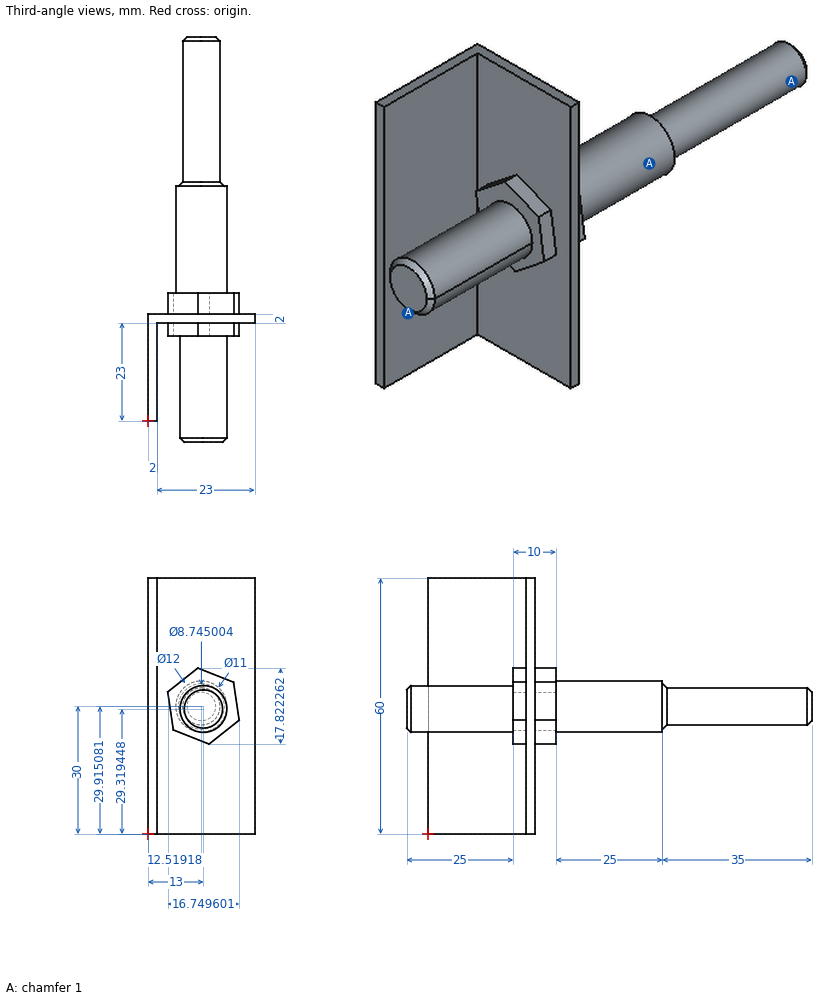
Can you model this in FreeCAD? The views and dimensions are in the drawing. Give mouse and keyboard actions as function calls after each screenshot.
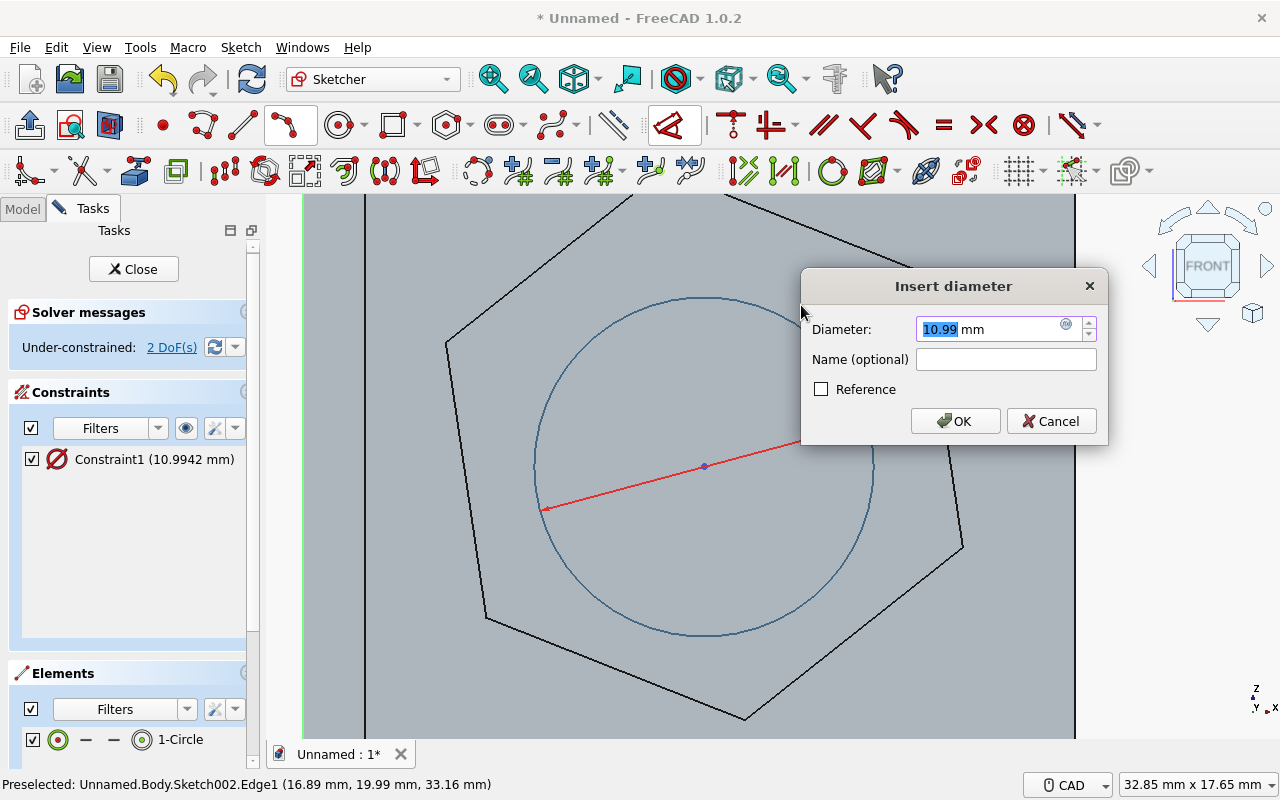
text(11)
key(Return)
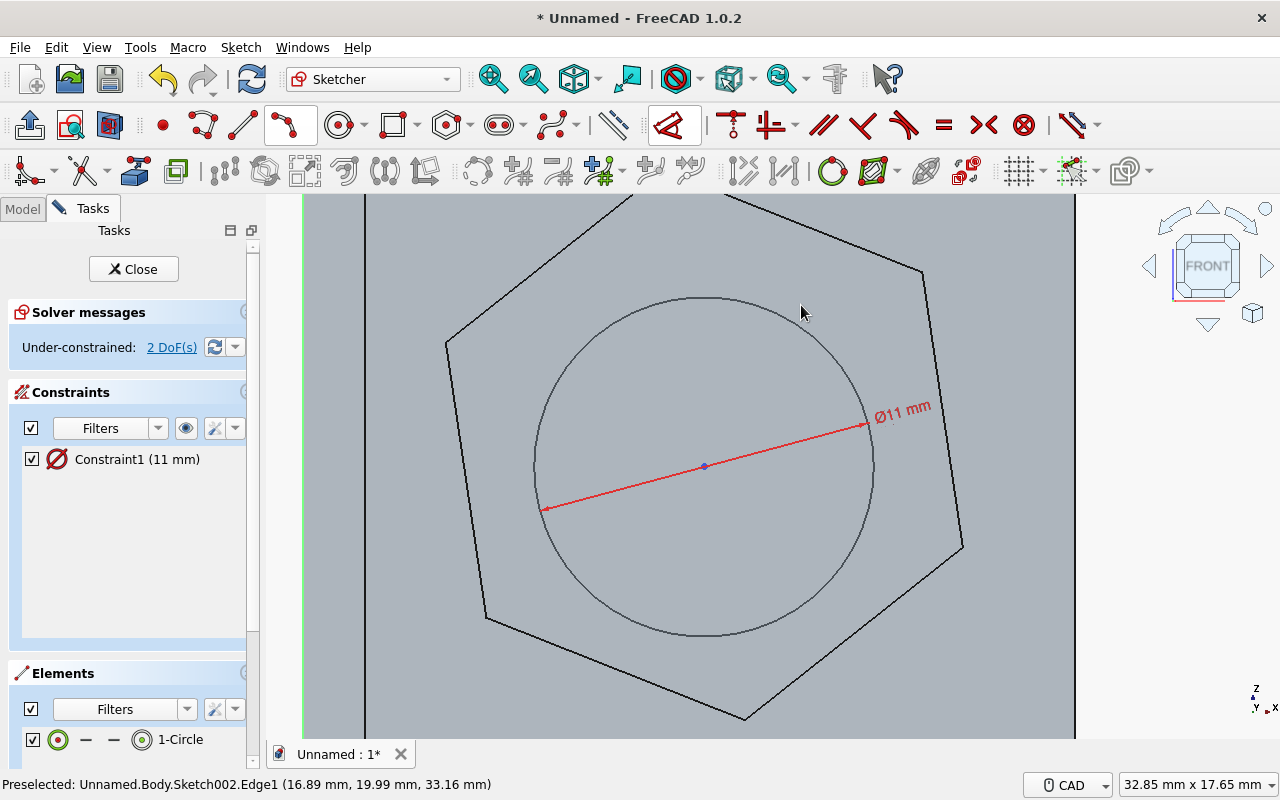
click(704, 467)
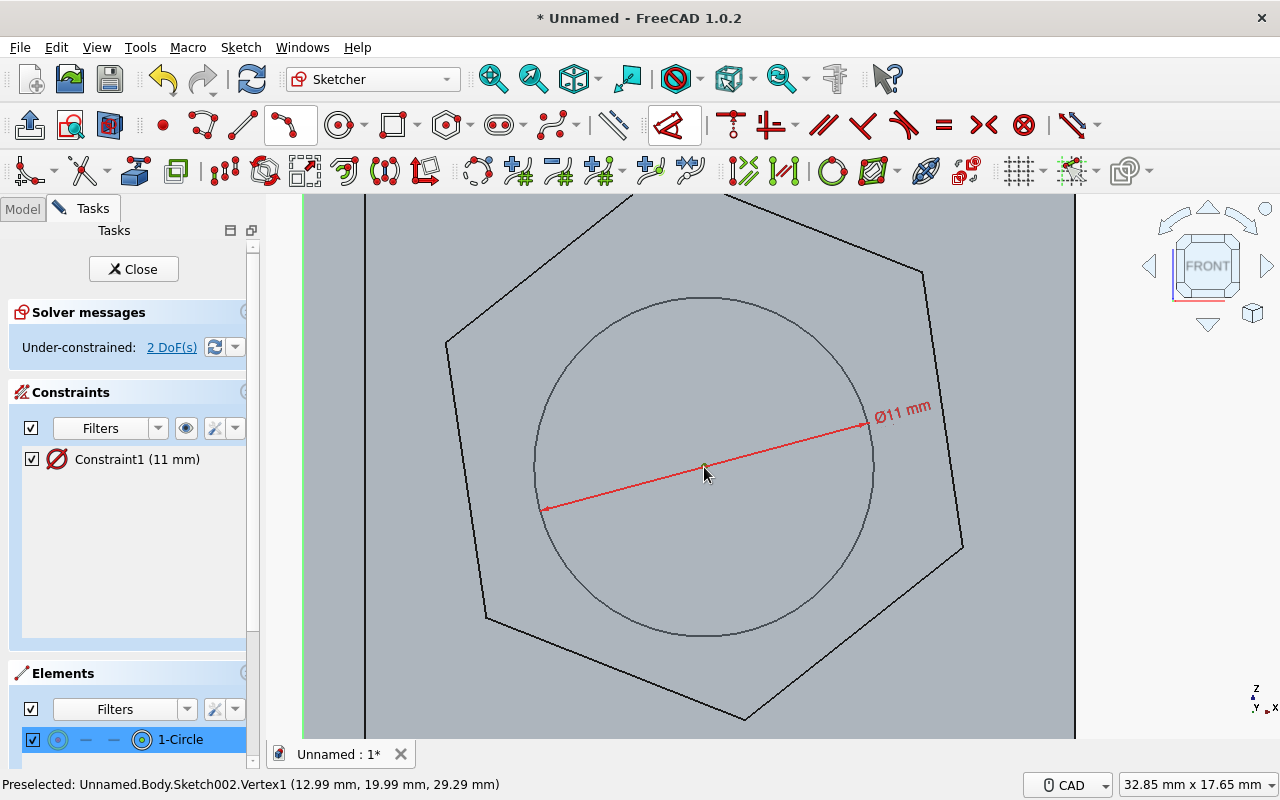
click(696, 126)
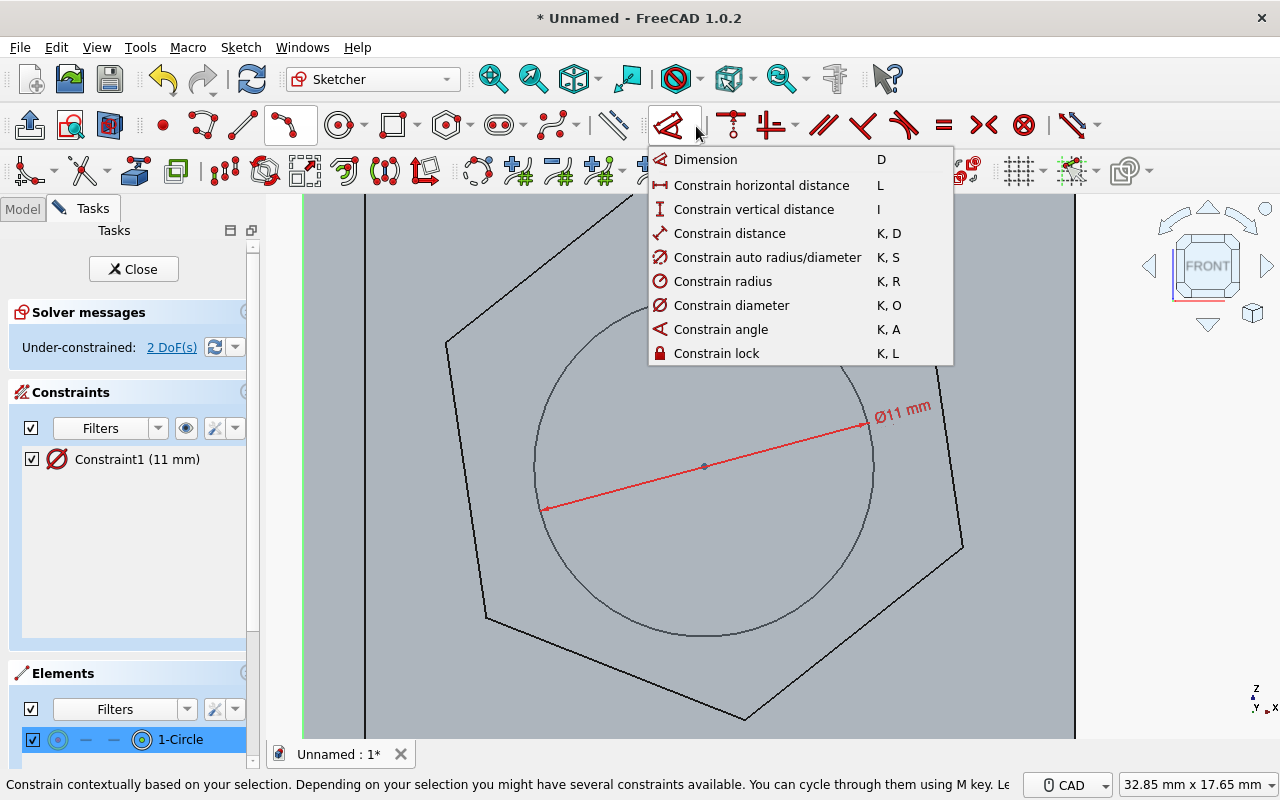
click(801, 185)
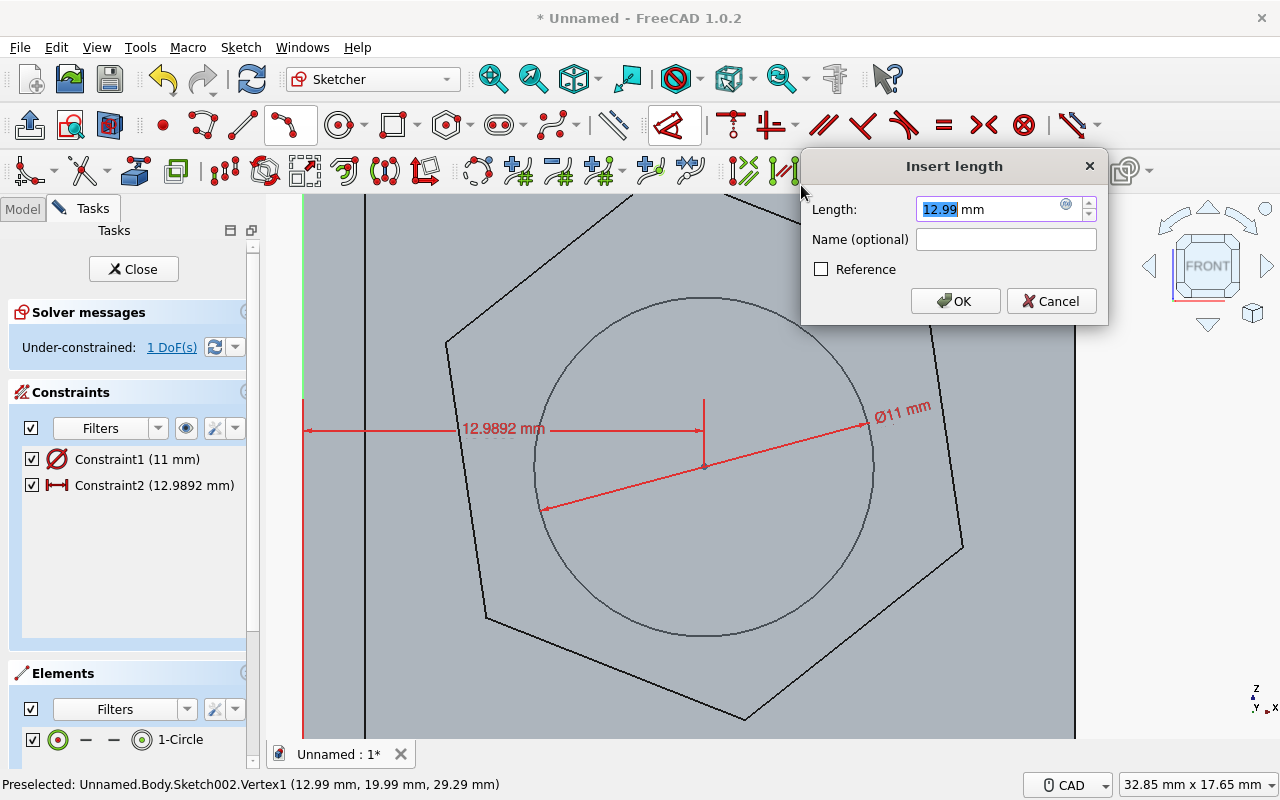
text(13)
key(Return)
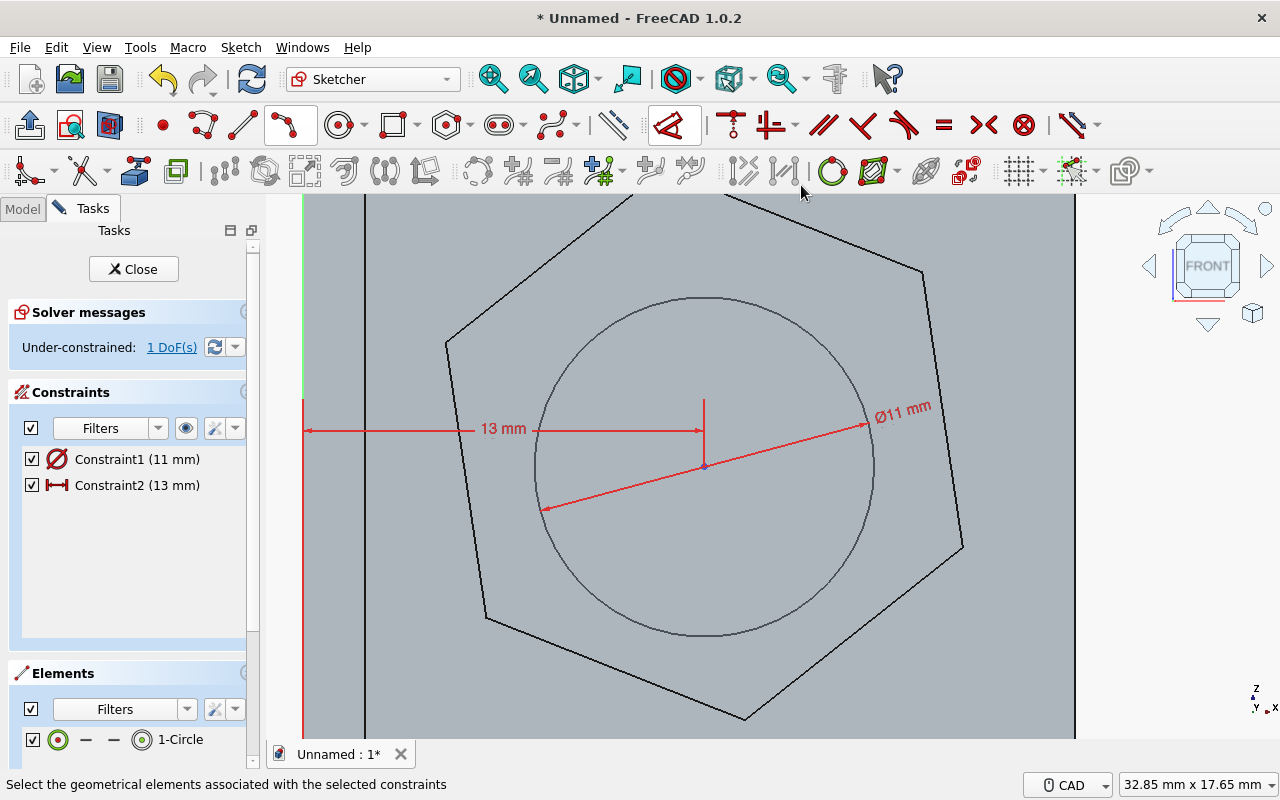
click(704, 467)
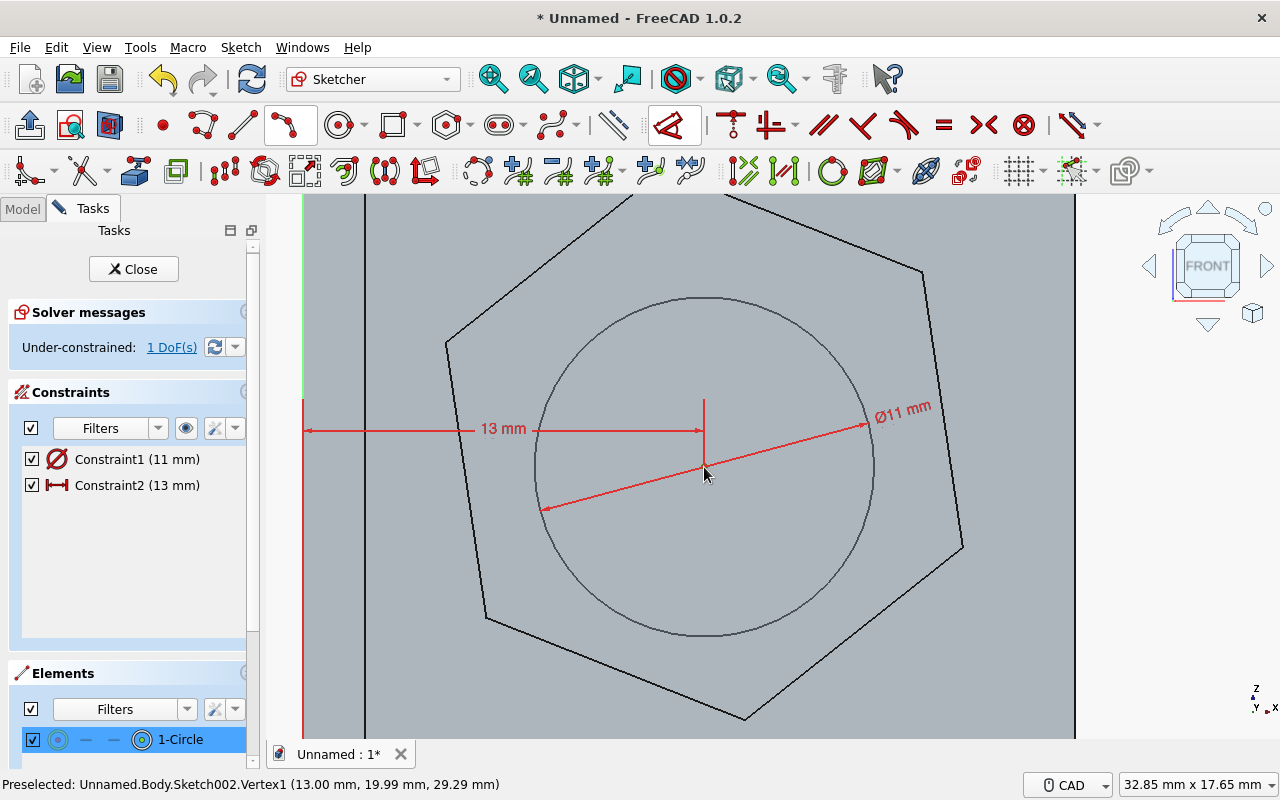
click(696, 126)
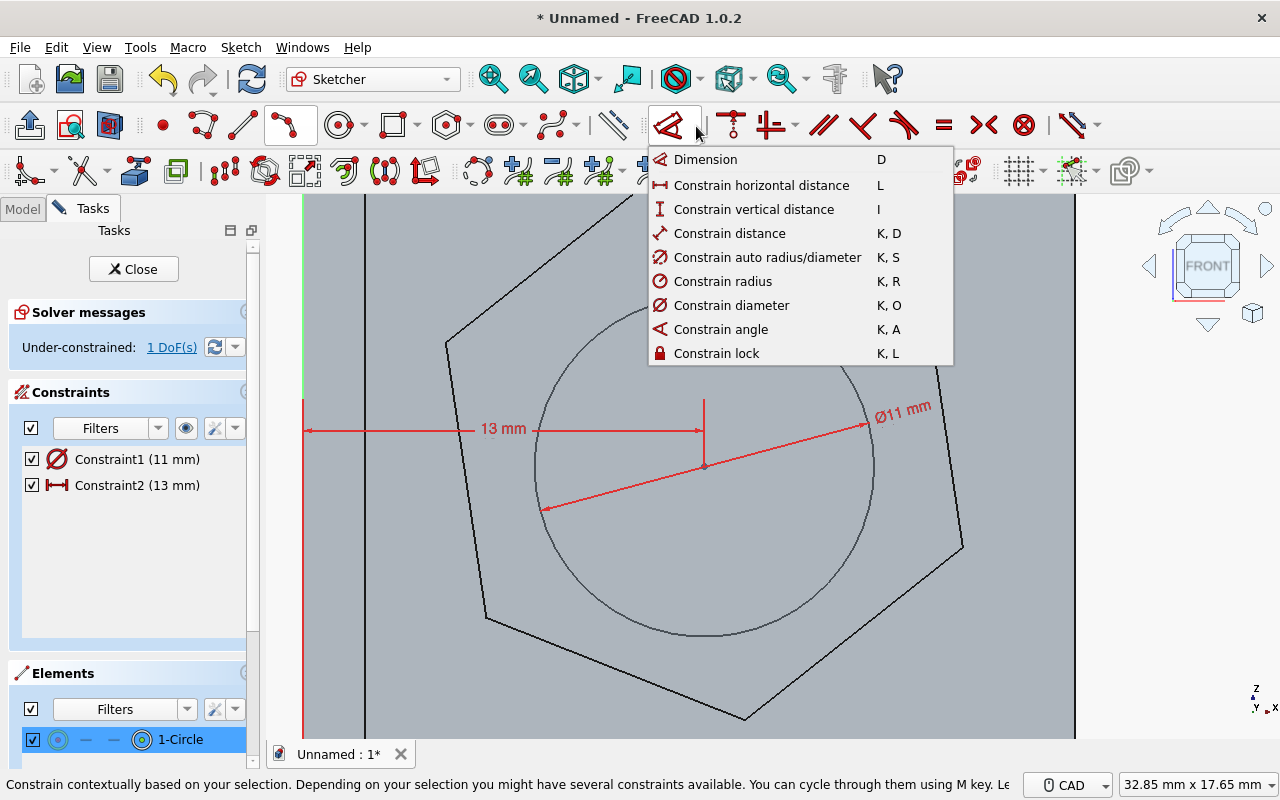
click(801, 209)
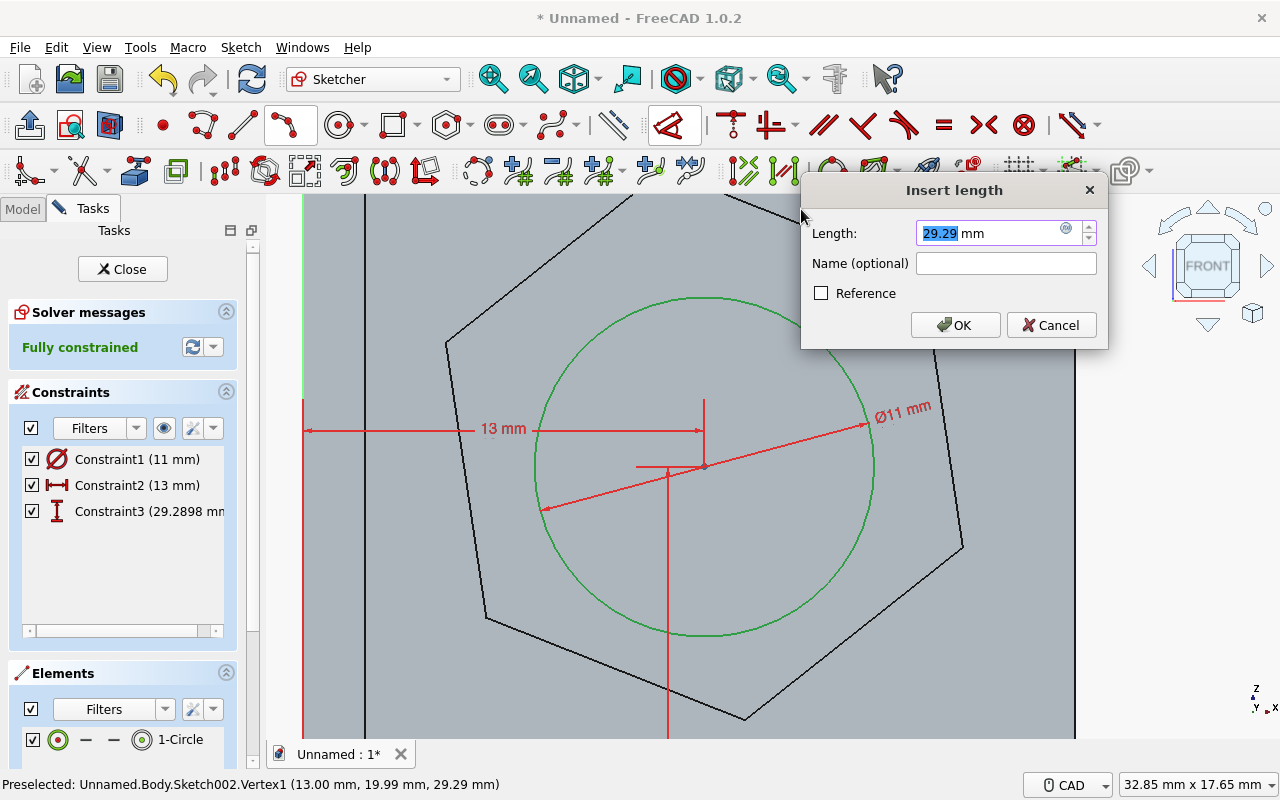
text(29.319448)
key(Return)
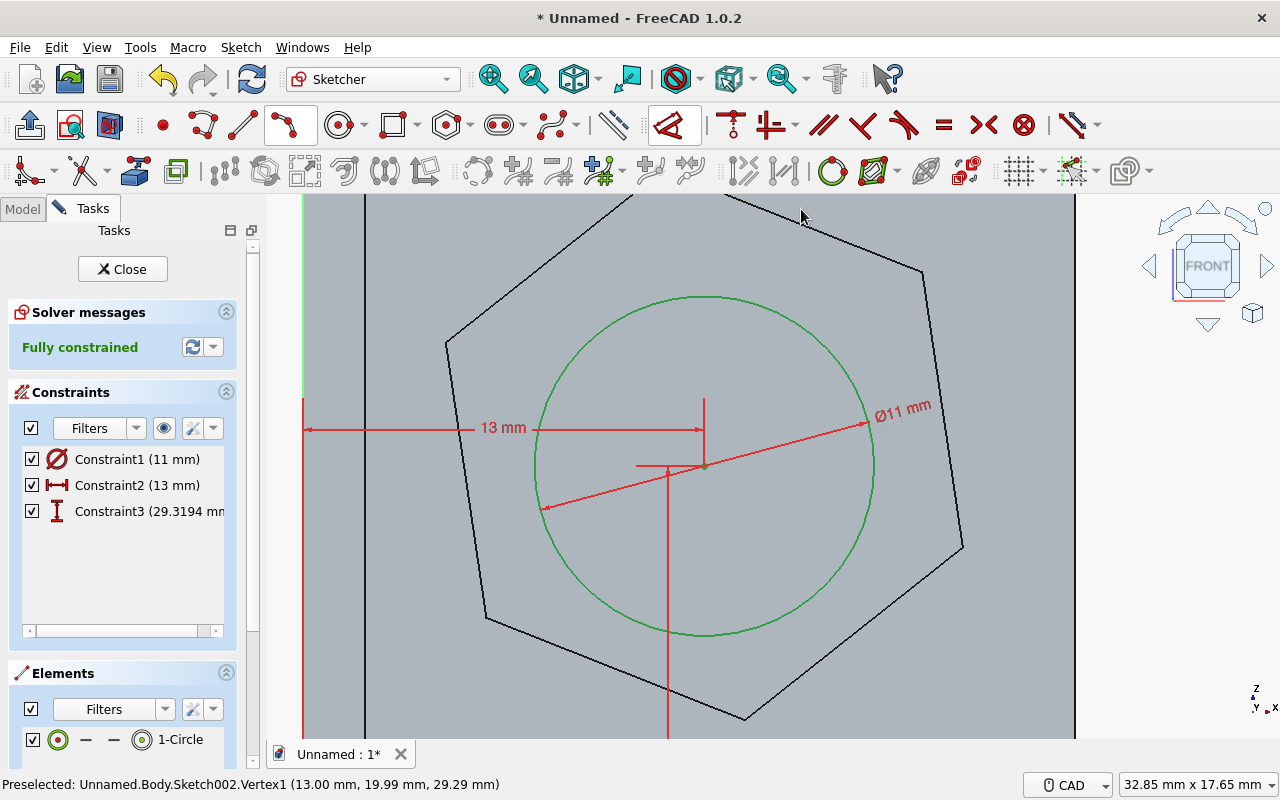
click(123, 269)